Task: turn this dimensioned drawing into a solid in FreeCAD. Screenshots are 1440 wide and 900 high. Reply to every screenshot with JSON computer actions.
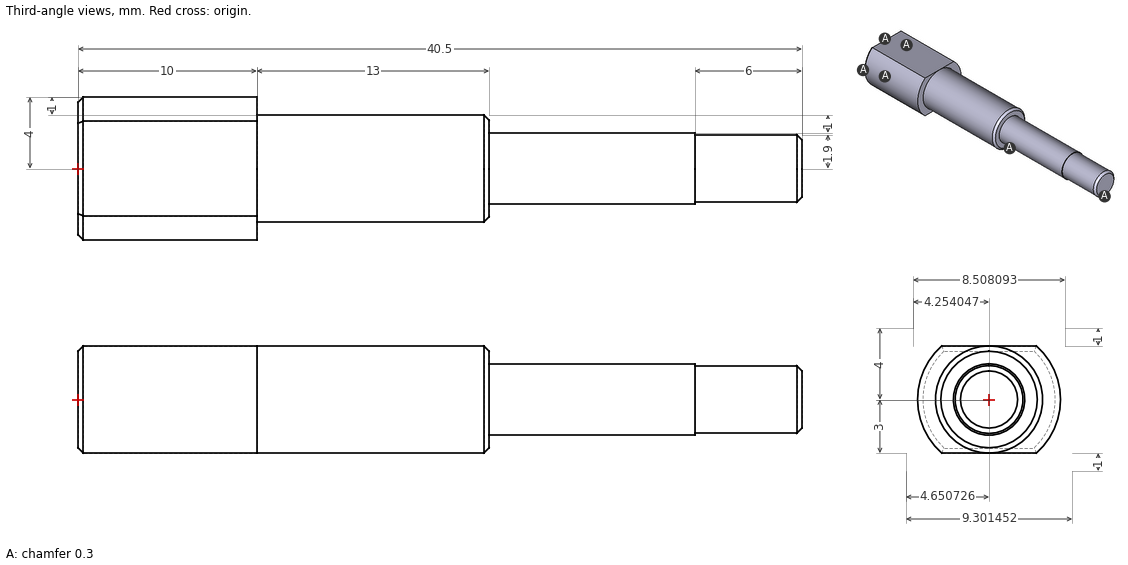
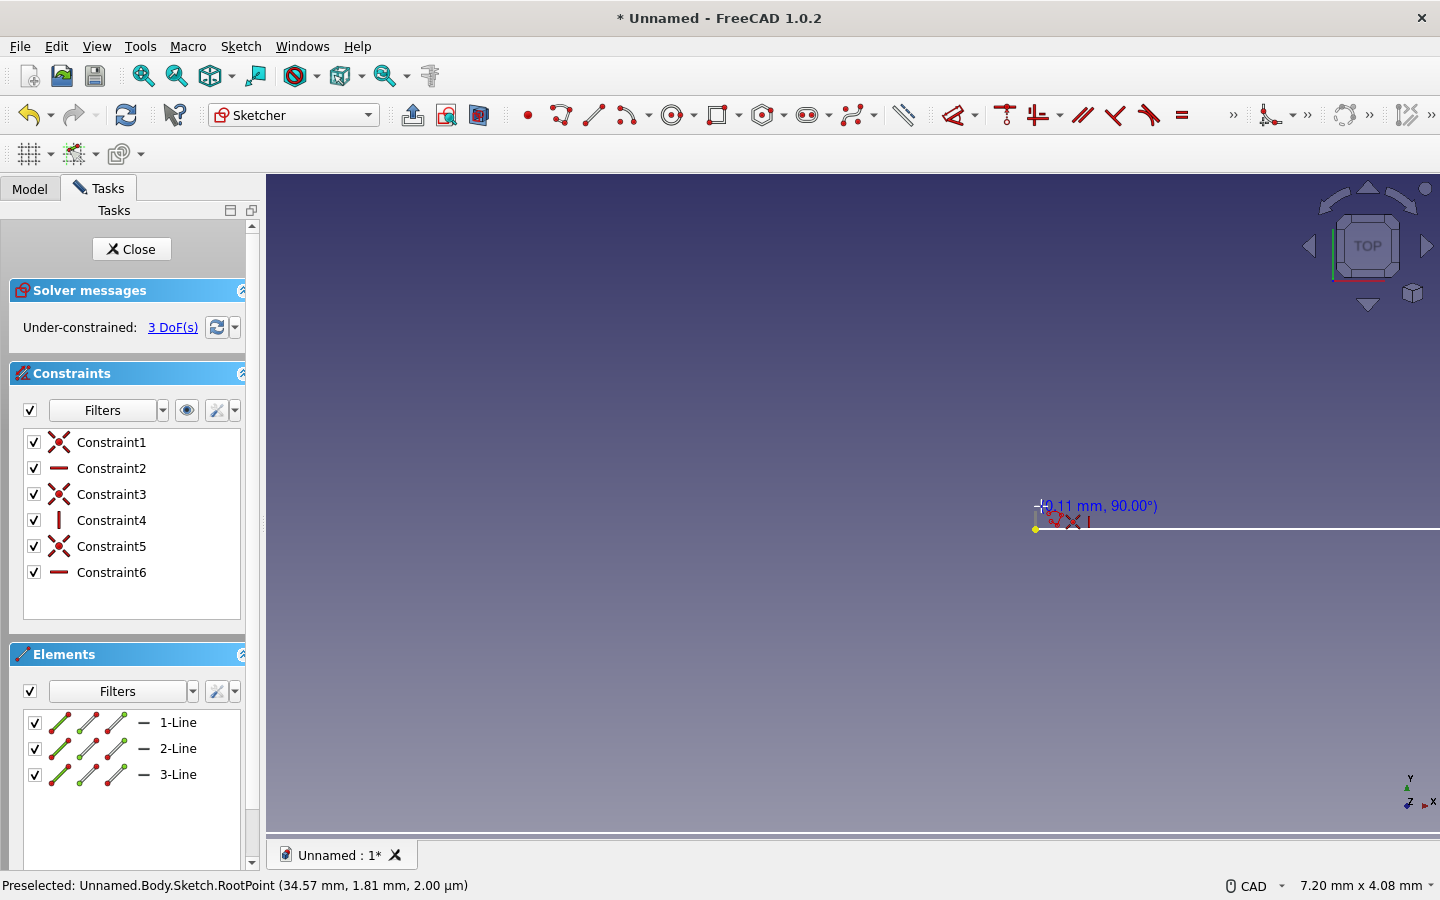
{"action": "left_click", "coordinate": [1036, 506]}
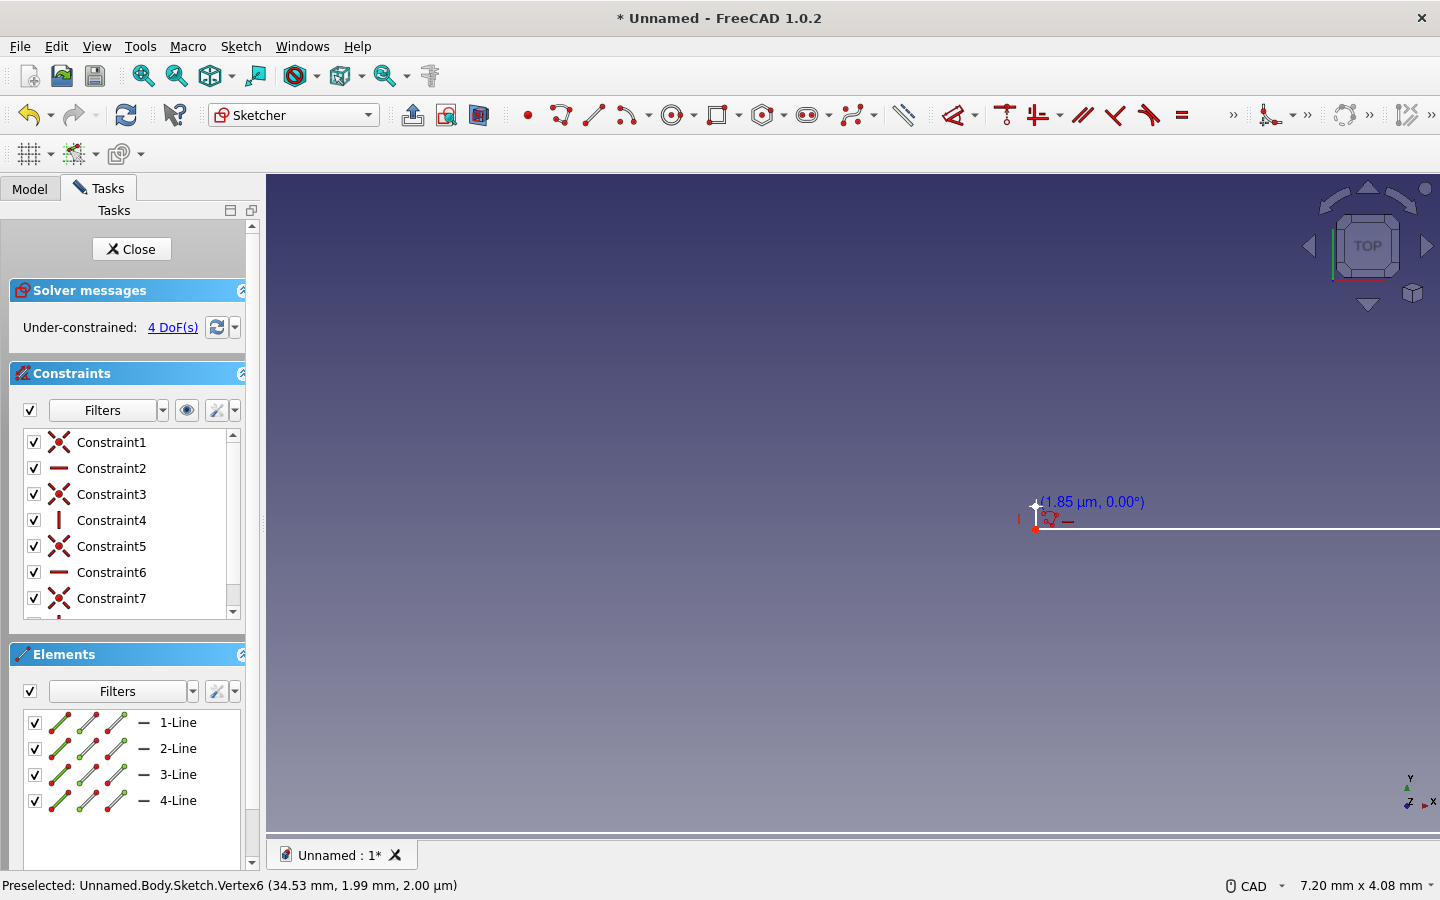
{"action": "scroll", "coordinate": [1043, 507], "scroll_direction": "down", "scroll_amount": 11}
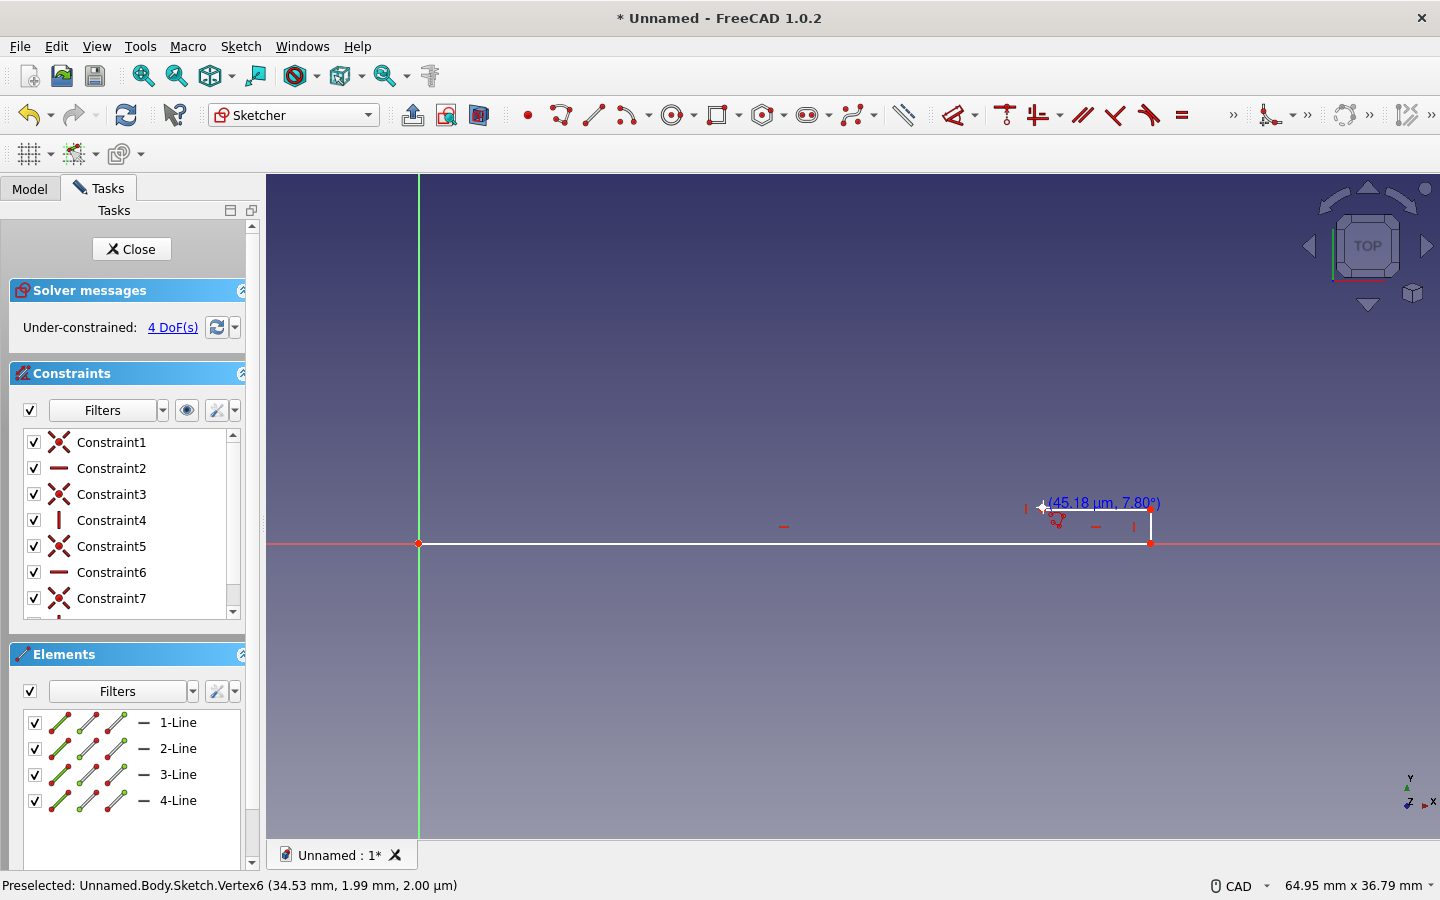
{"action": "left_click", "coordinate": [835, 507]}
{"action": "left_click", "coordinate": [835, 489]}
{"action": "left_click", "coordinate": [600, 489]}
{"action": "left_click", "coordinate": [600, 471]}
{"action": "left_click", "coordinate": [428, 471]}
{"action": "left_click", "coordinate": [419, 544]}
{"action": "key", "text": "Escape"}
{"action": "key", "text": "Escape"}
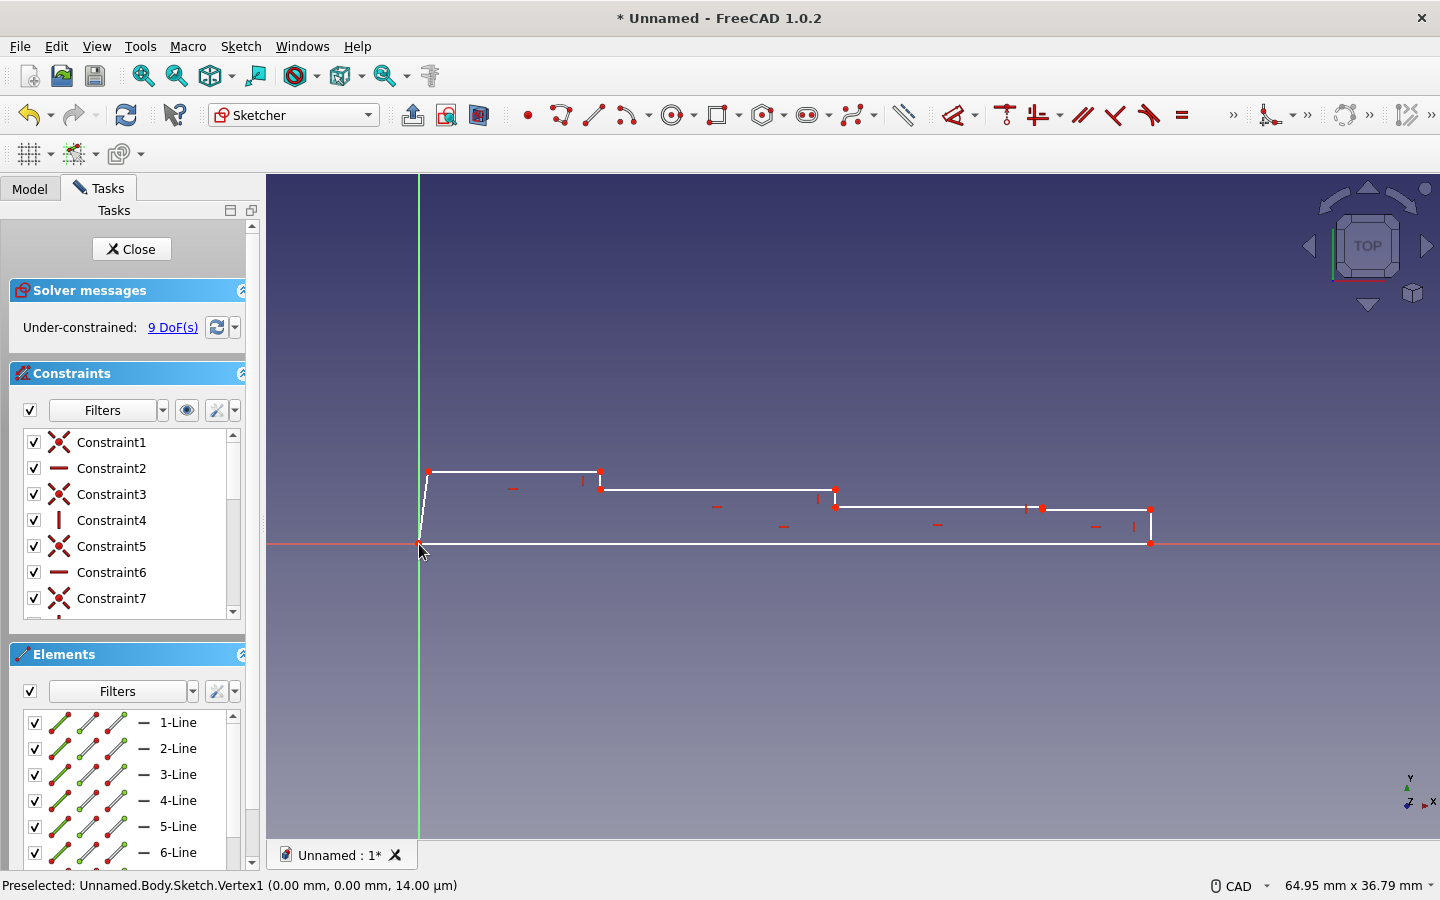
{"action": "left_click", "coordinate": [422, 522]}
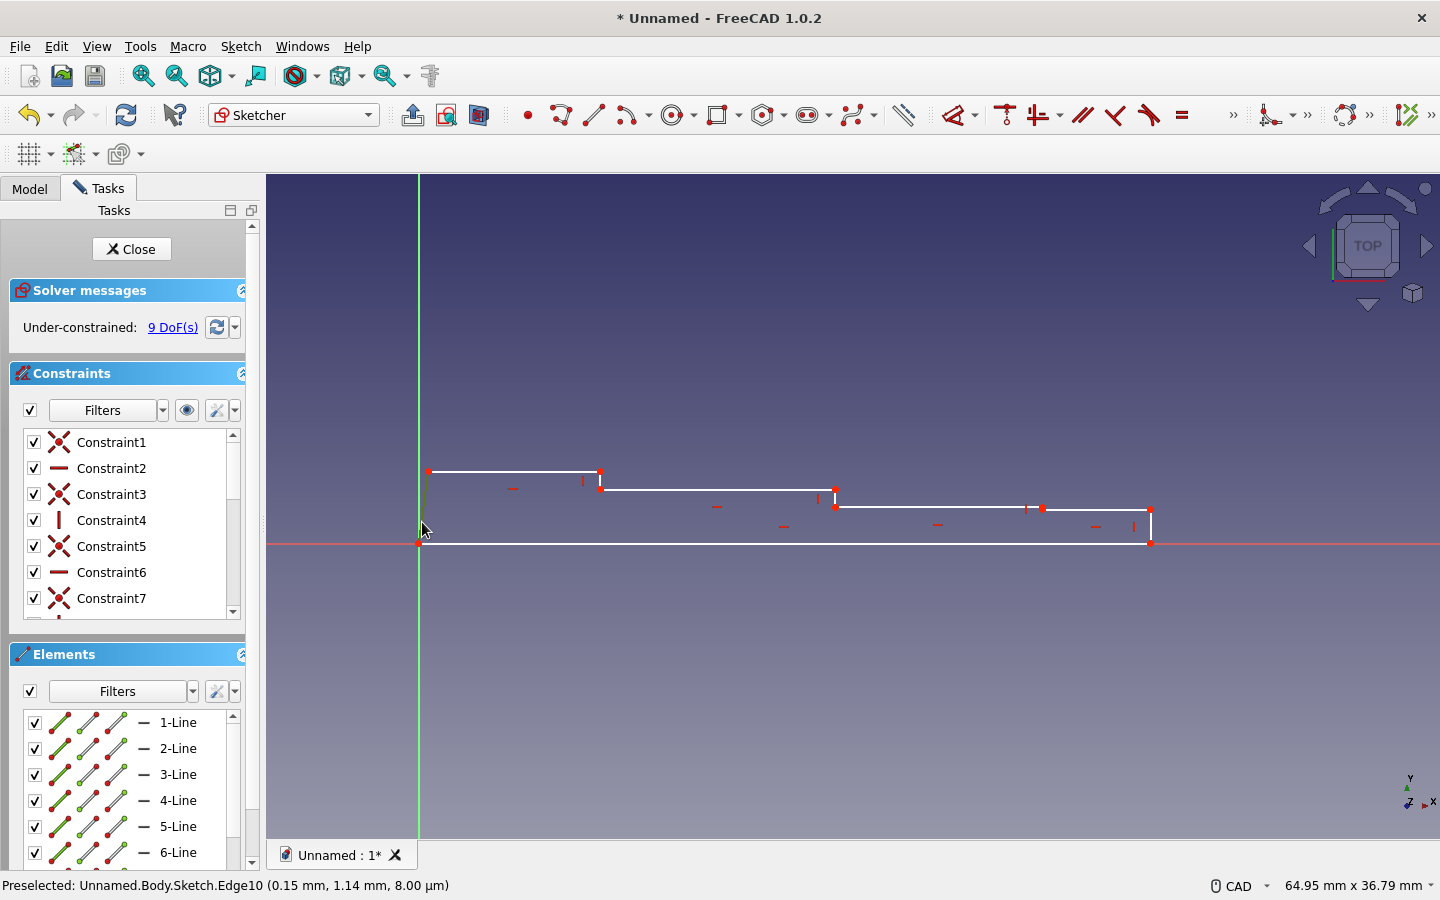
{"action": "key", "text": "v"}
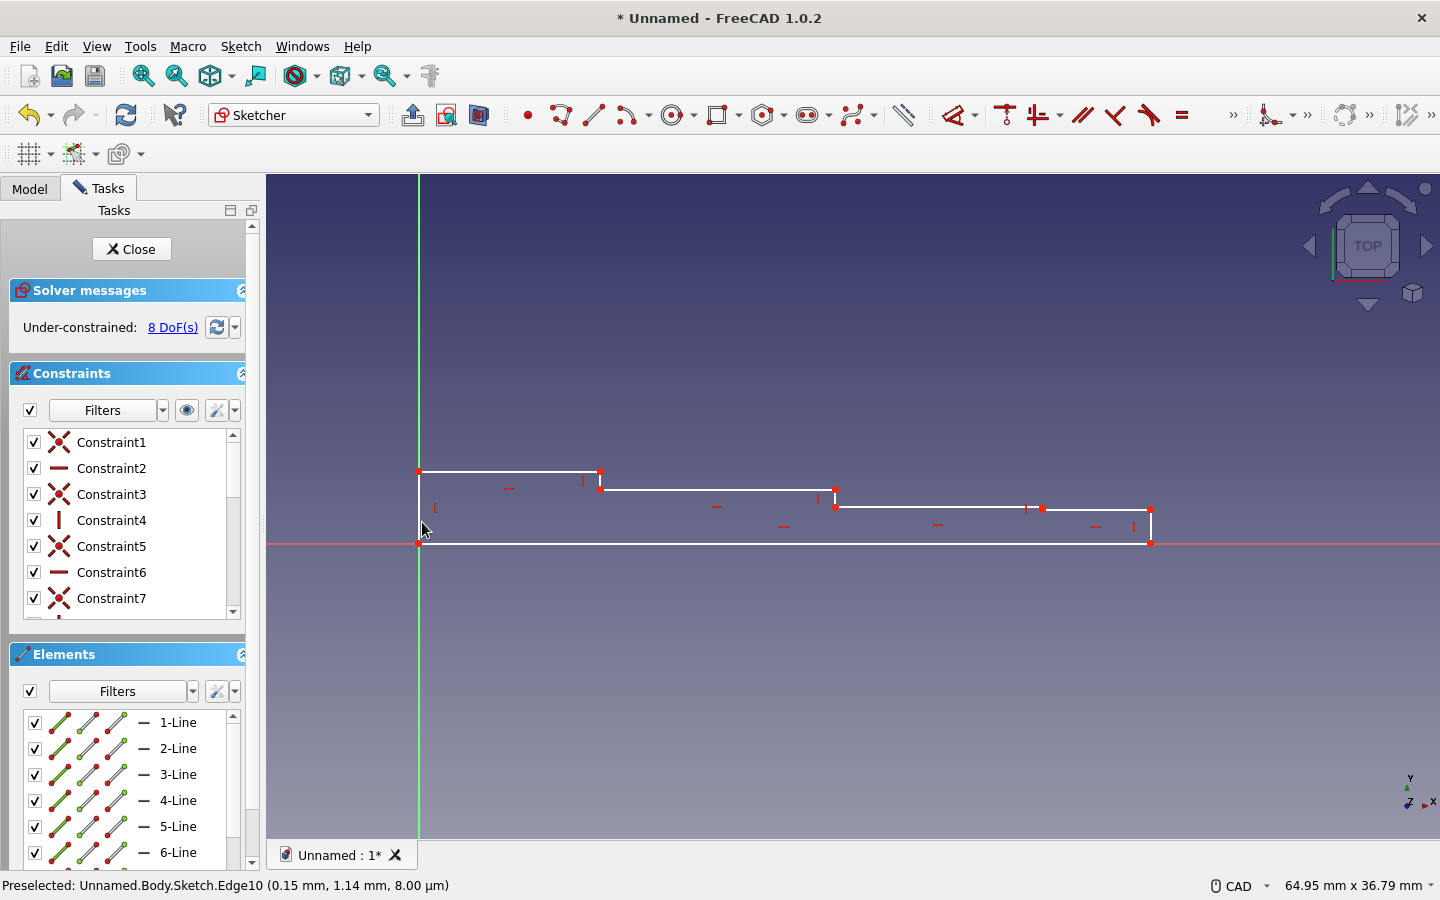
{"action": "key", "text": "d"}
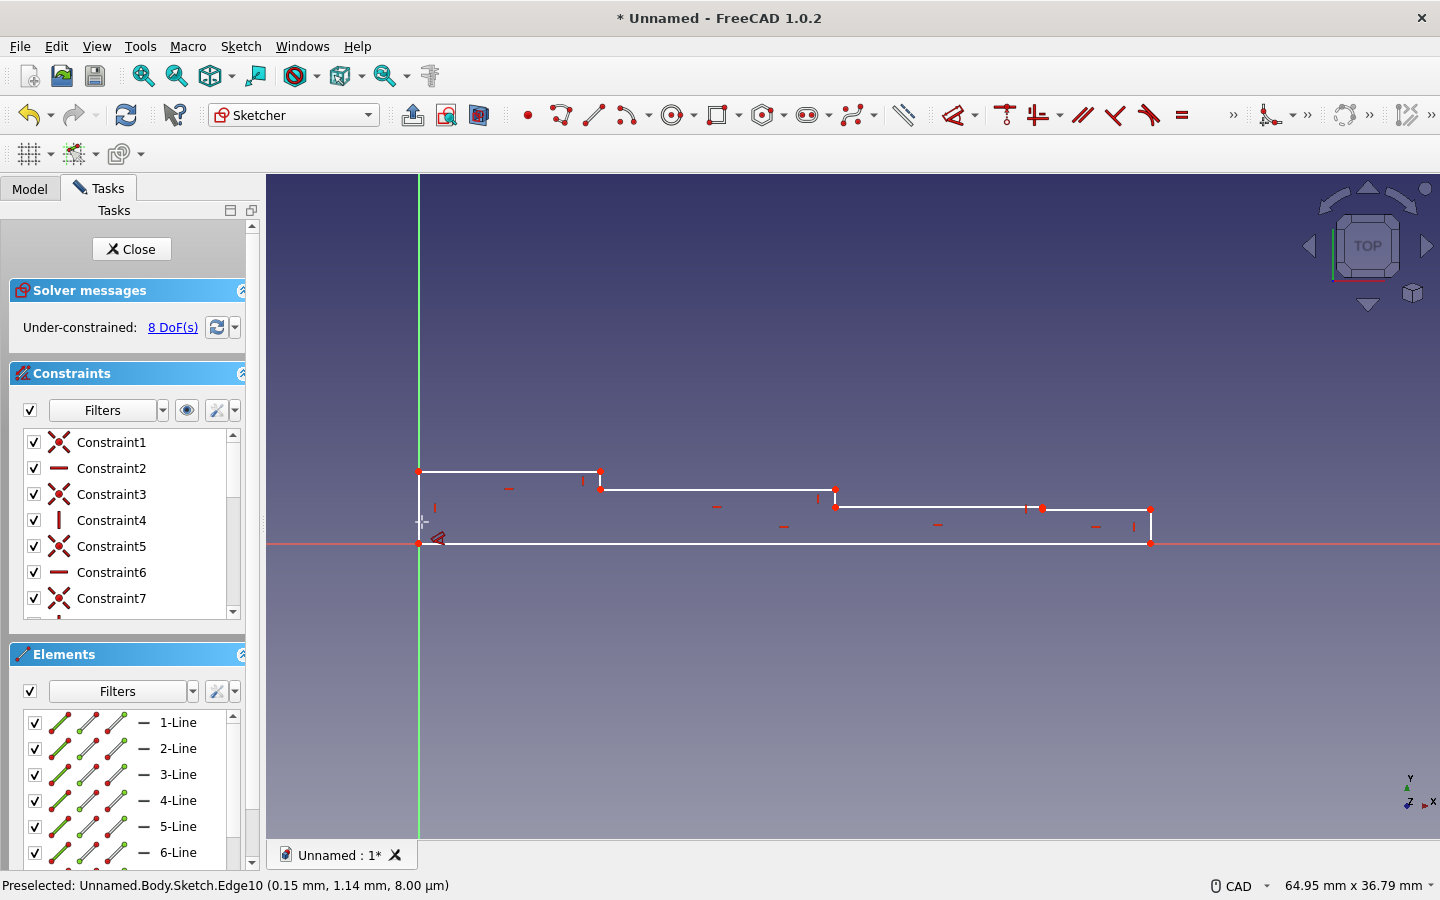
{"action": "left_click", "coordinate": [1118, 510]}
{"action": "left_click", "coordinate": [1097, 476]}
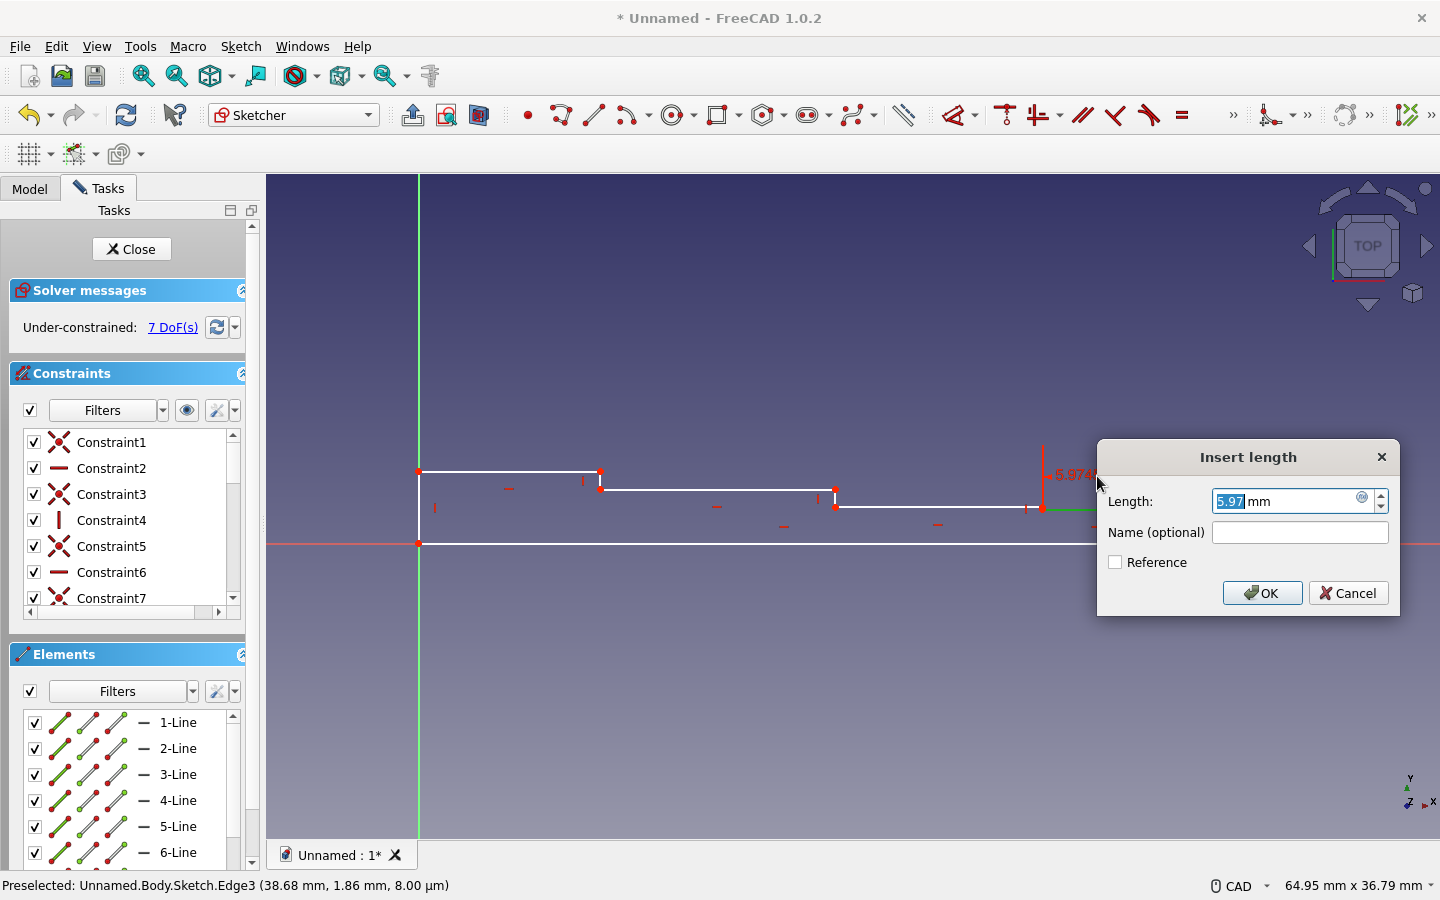
{"action": "type", "text": "6"}
{"action": "key", "text": "Return"}